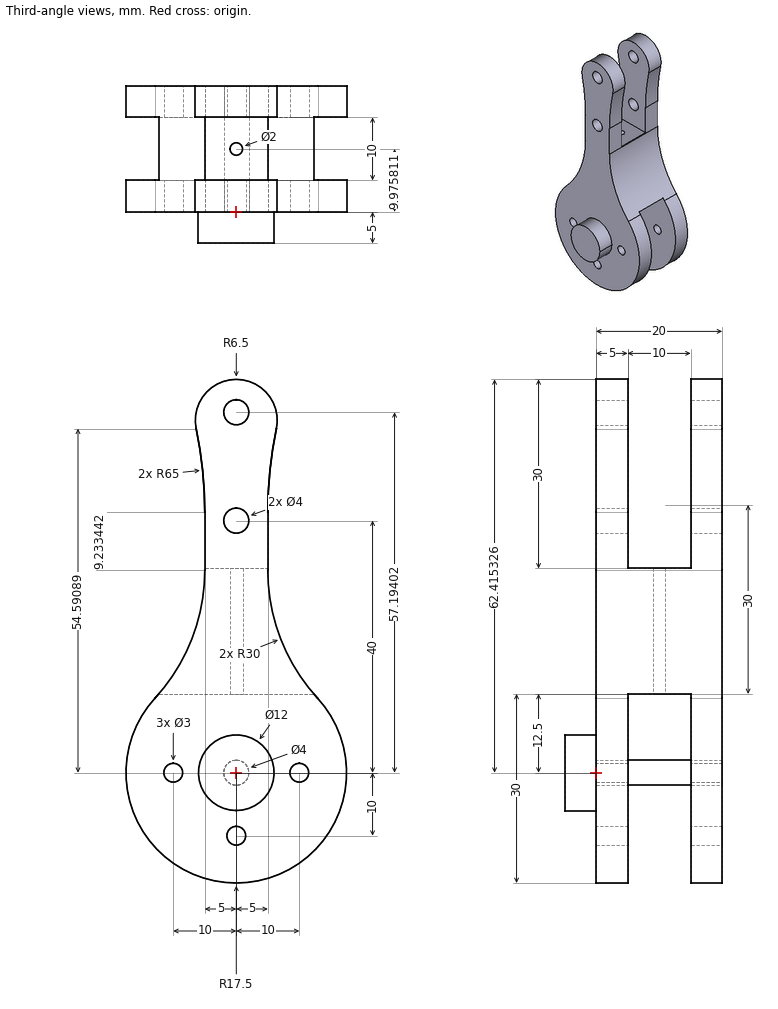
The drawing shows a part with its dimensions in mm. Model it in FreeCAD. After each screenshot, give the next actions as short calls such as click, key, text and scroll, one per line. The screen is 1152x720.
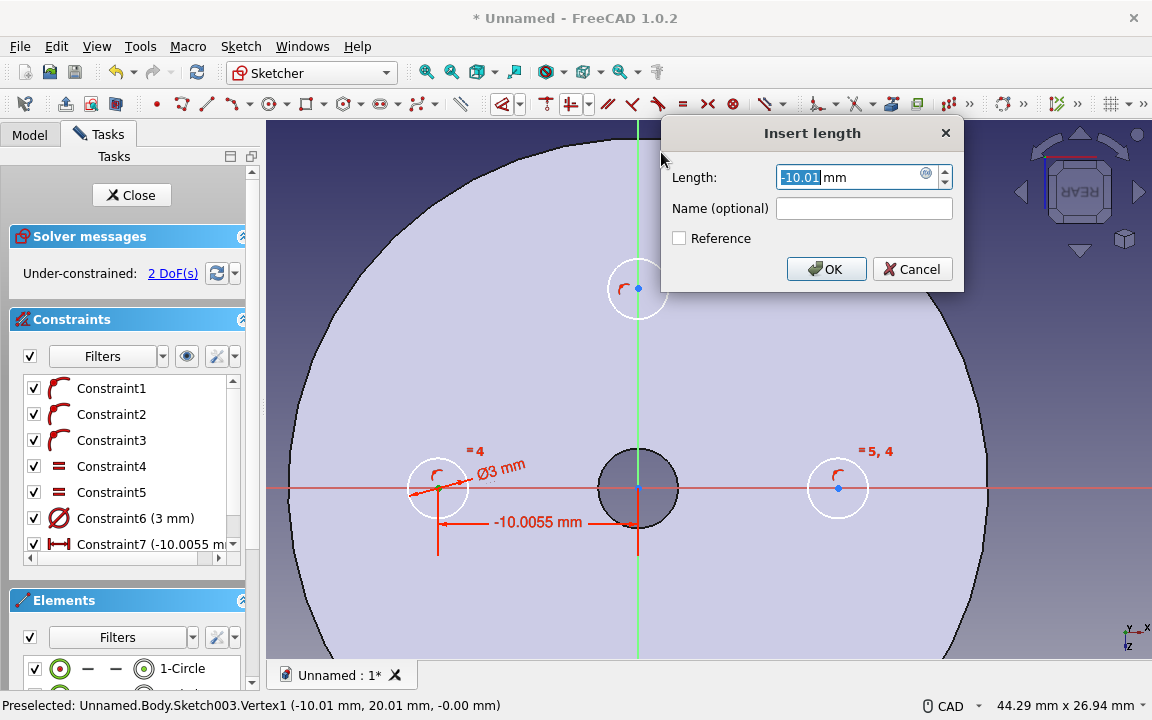
text(-10)
key(Return)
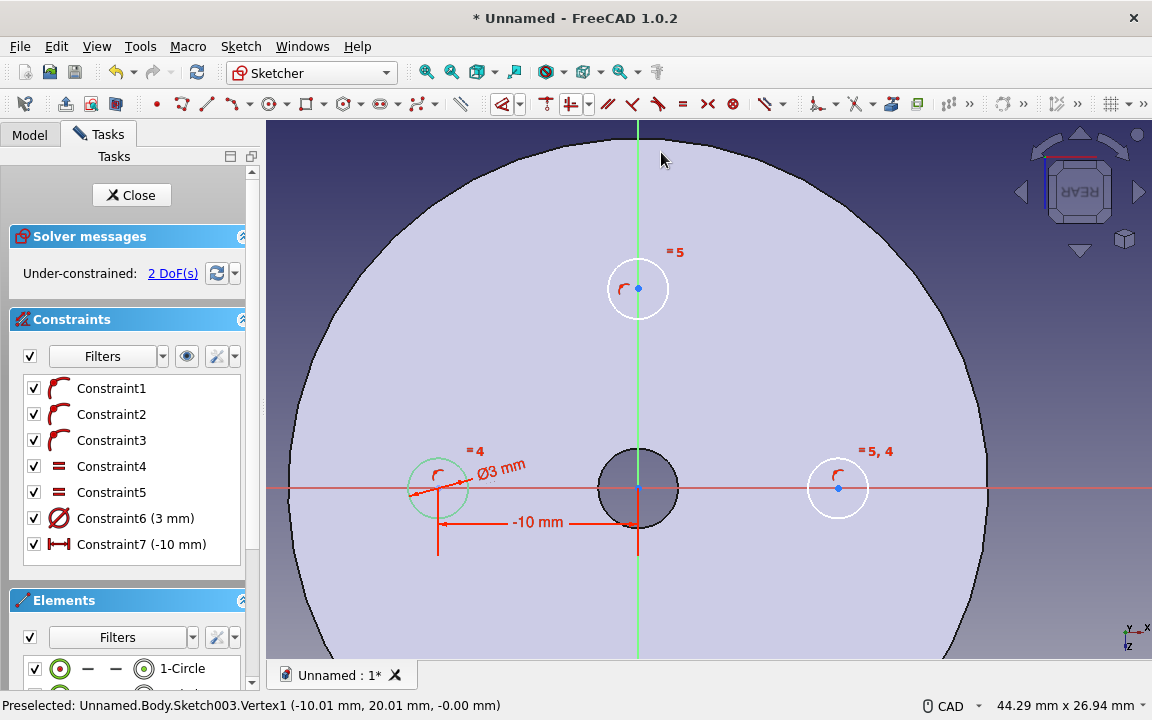
click(838, 488)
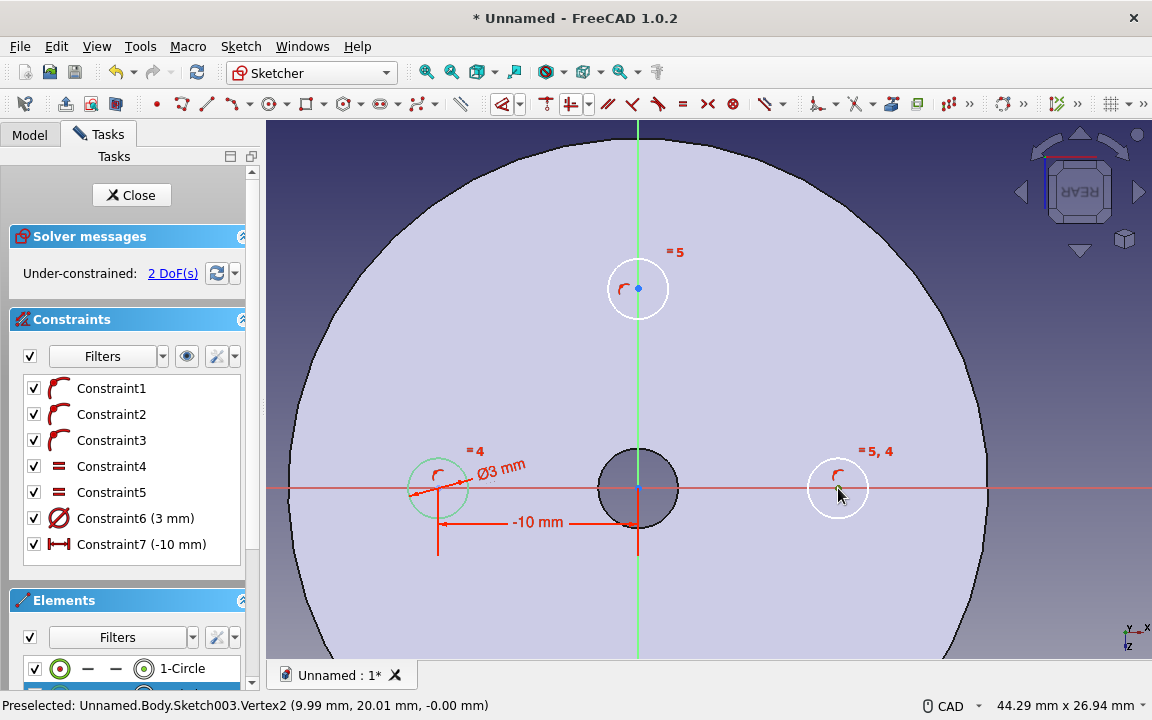
click(520, 104)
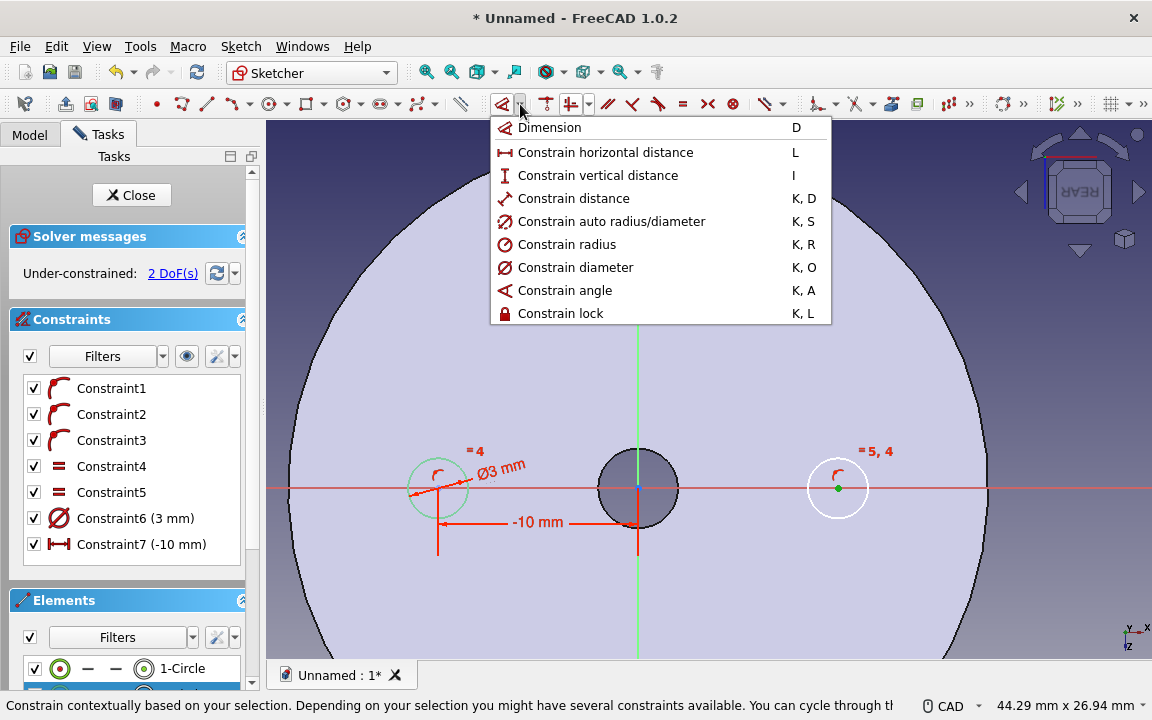
click(661, 152)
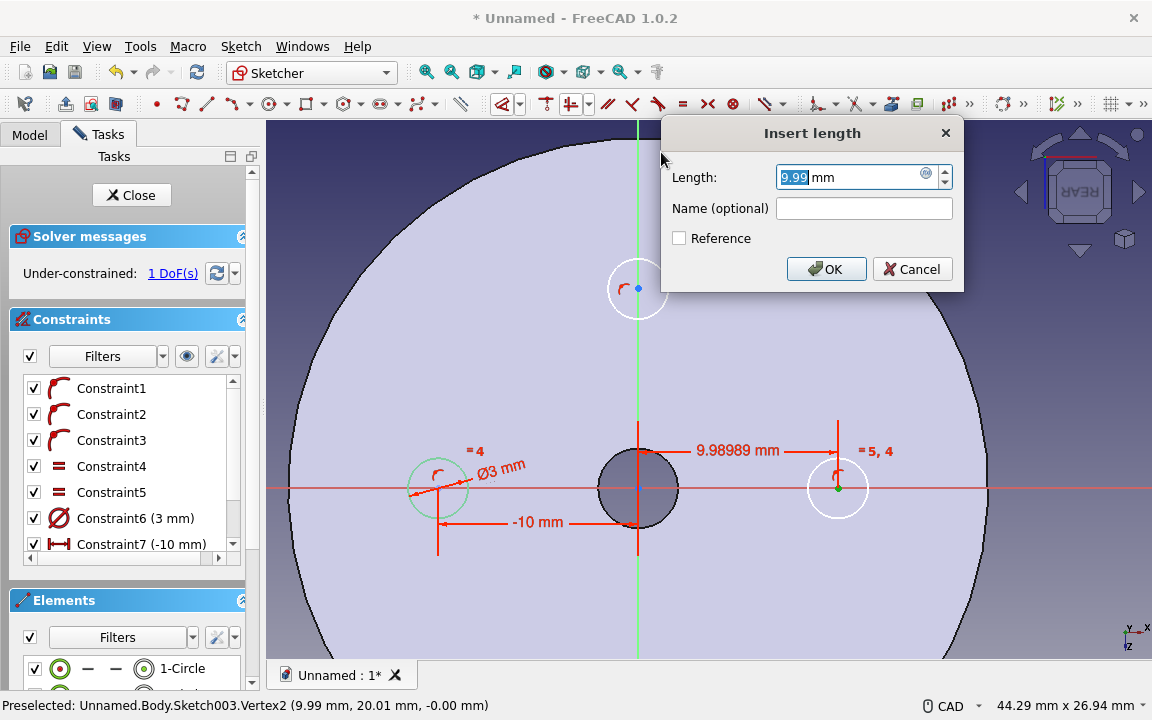
text(10)
key(Return)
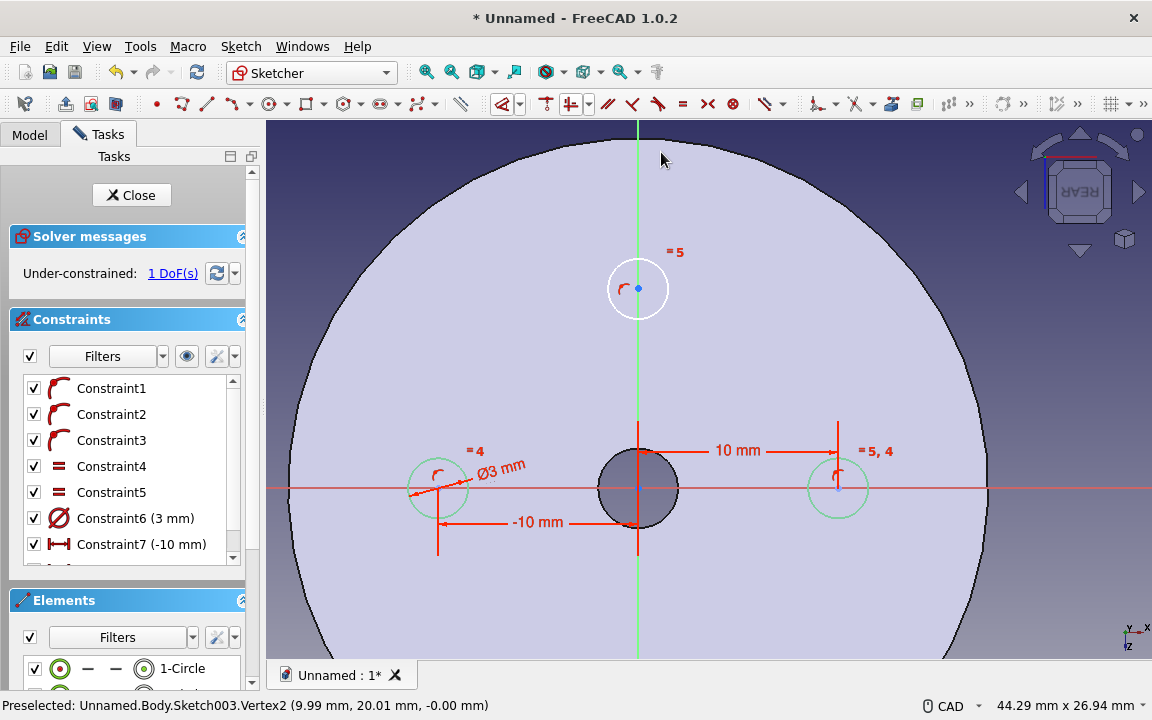
click(638, 289)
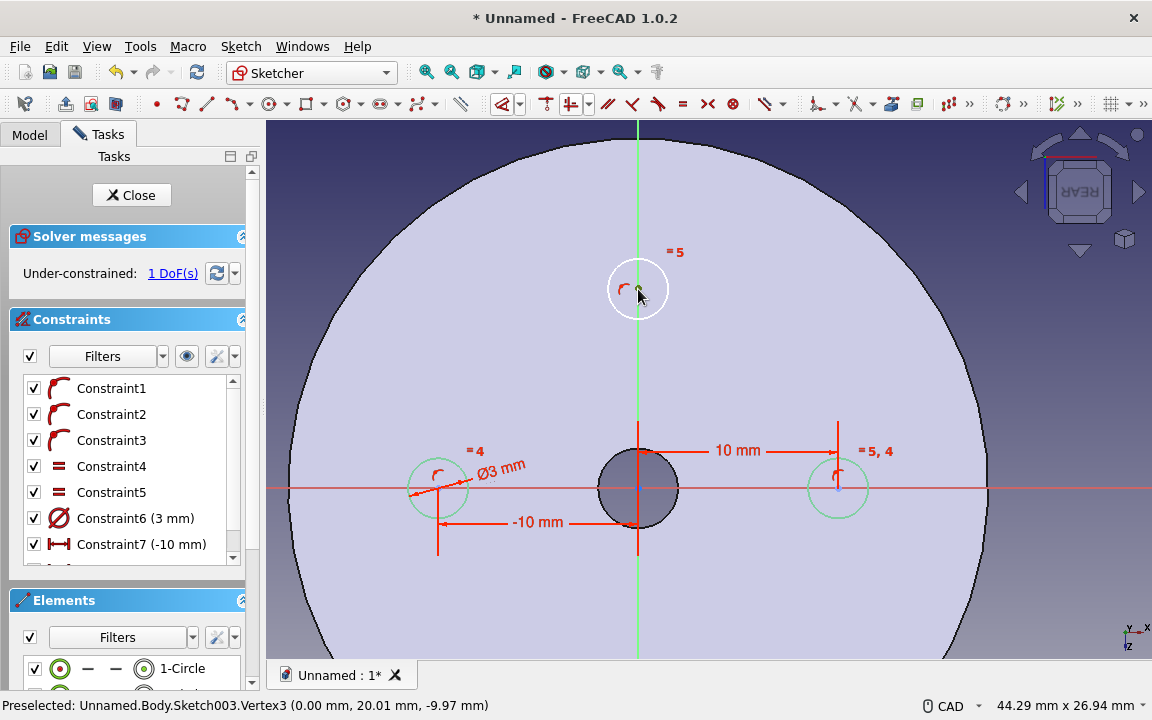
click(520, 104)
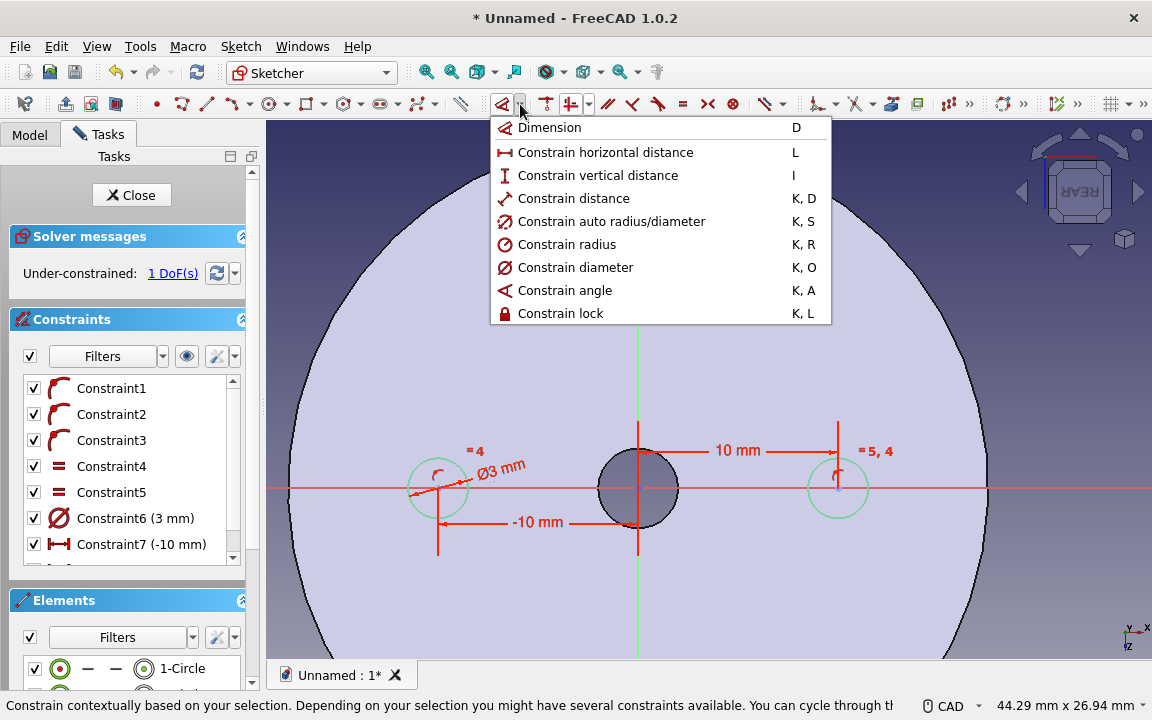
click(661, 176)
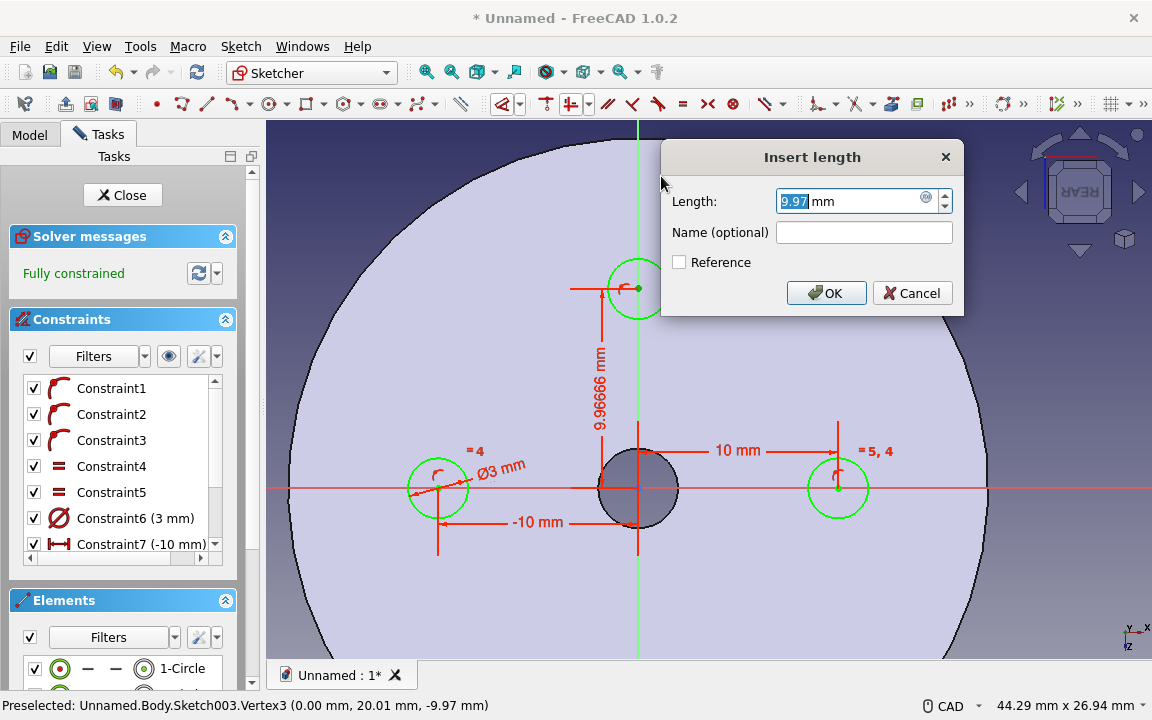
text(10)
key(Return)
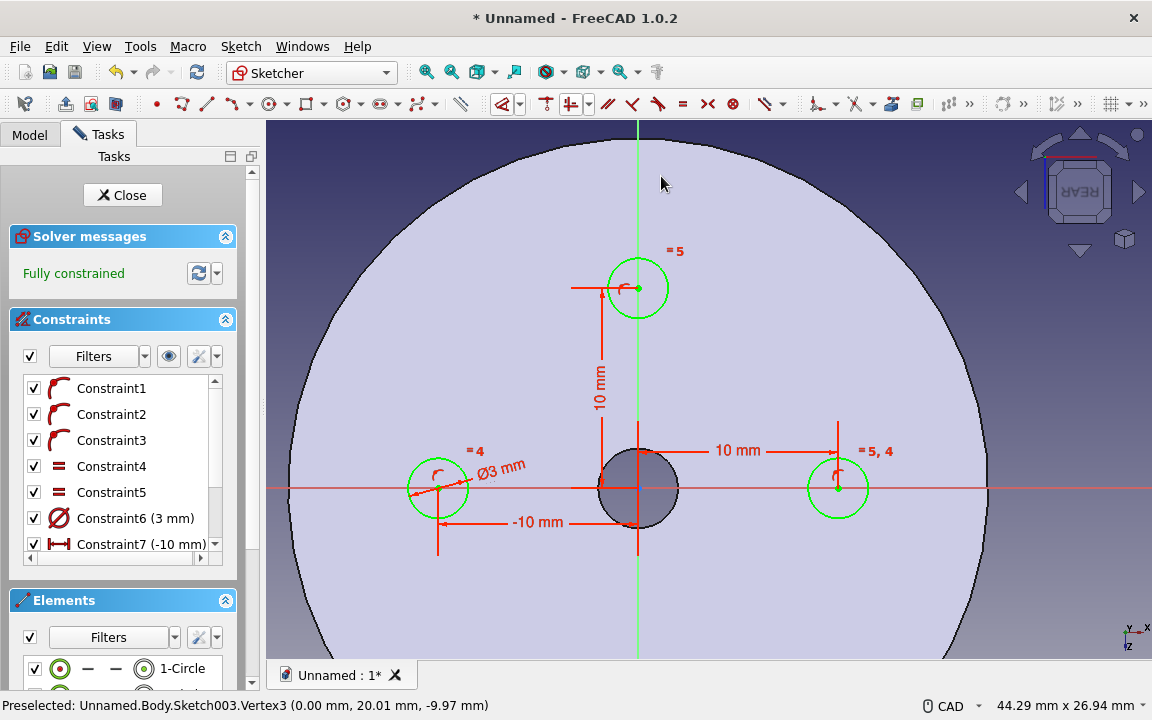
click(123, 195)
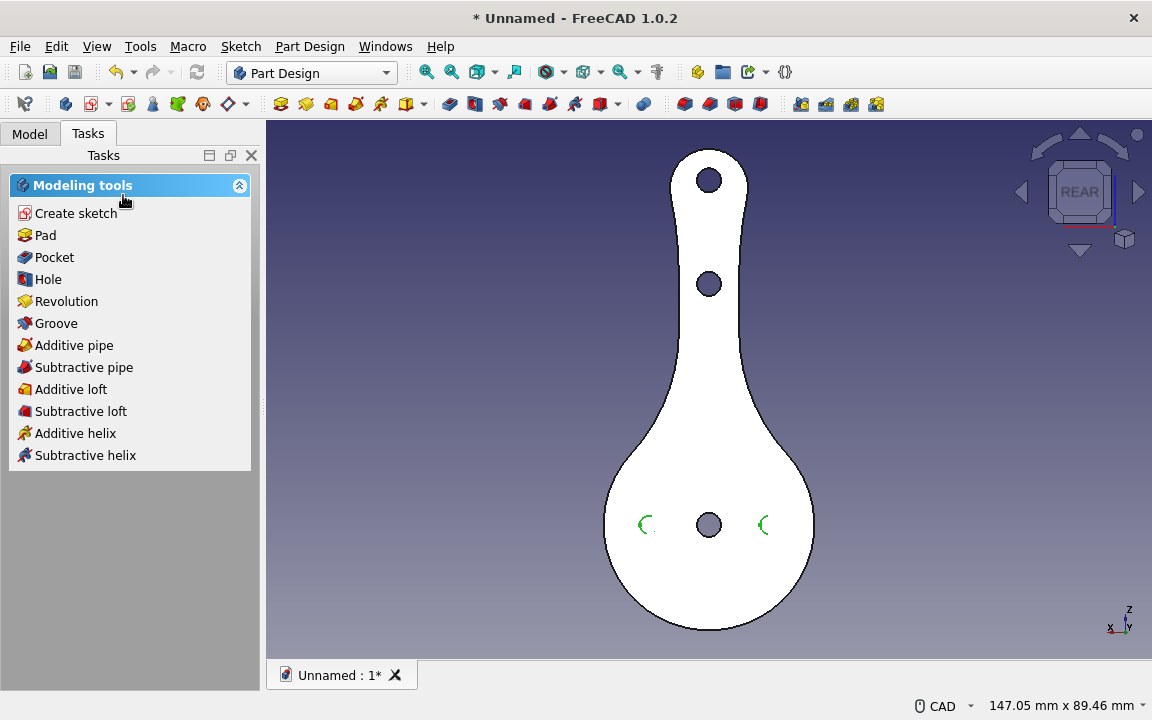
click(450, 104)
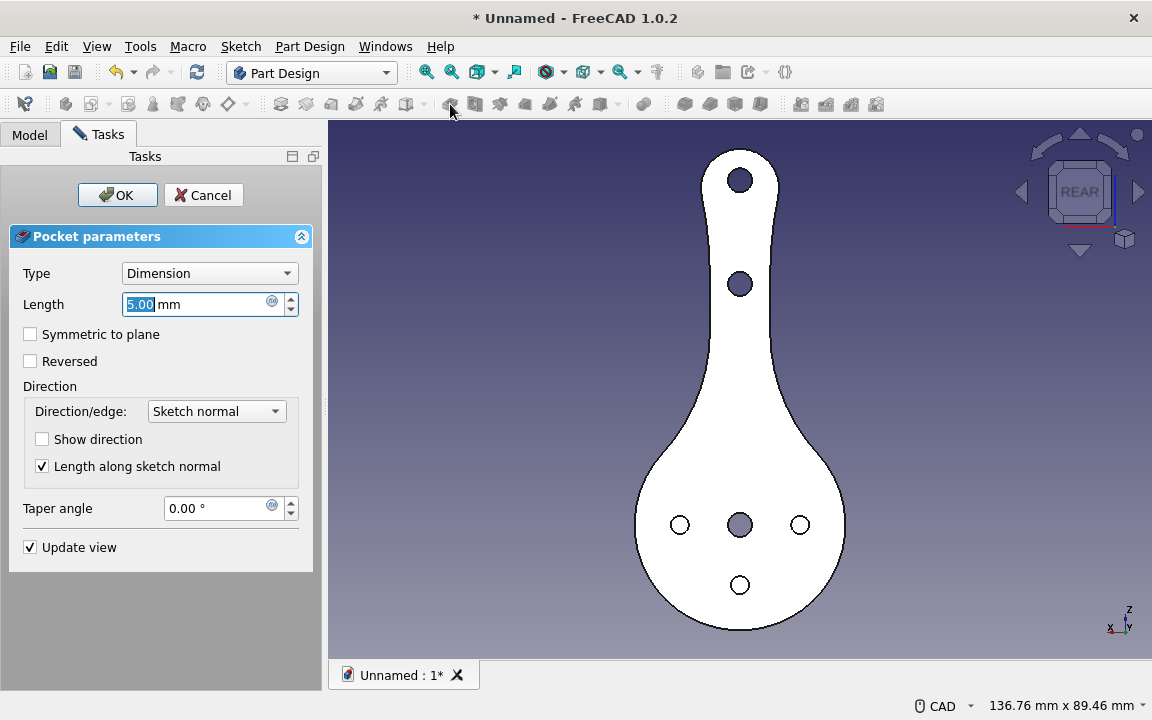
click(210, 274)